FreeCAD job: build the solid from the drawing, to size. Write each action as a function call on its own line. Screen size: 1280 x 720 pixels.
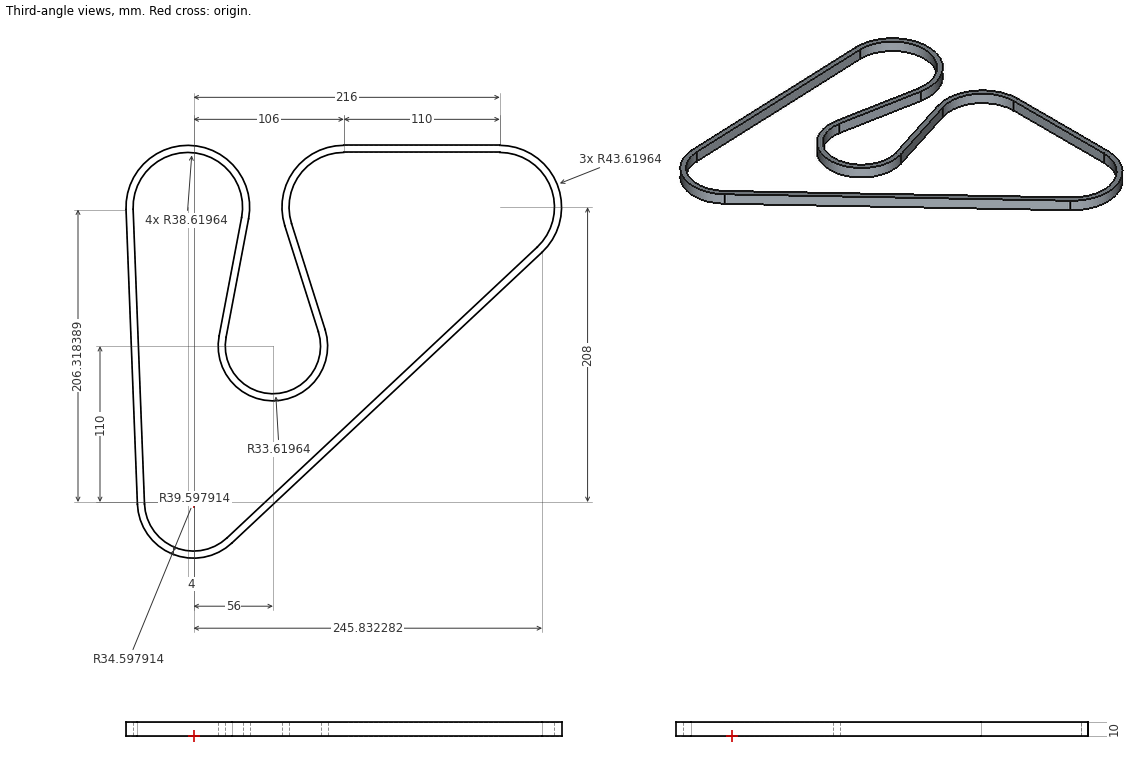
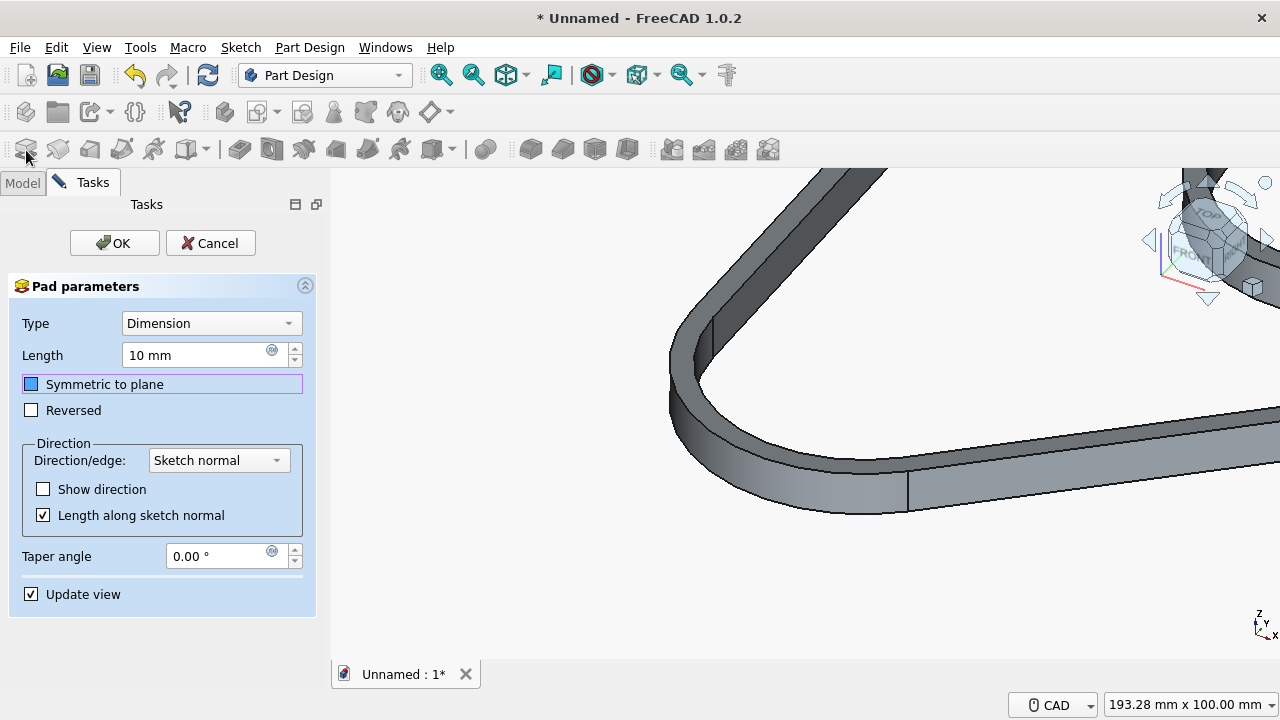
click(115, 243)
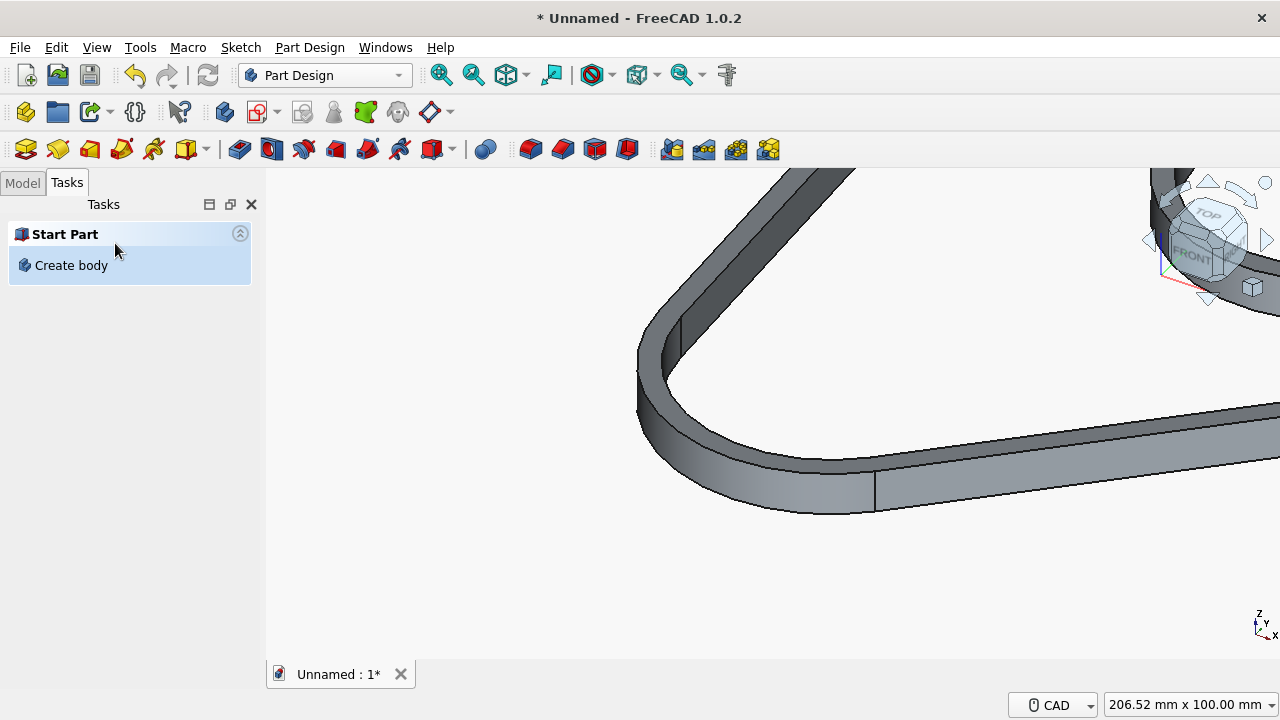
key(0)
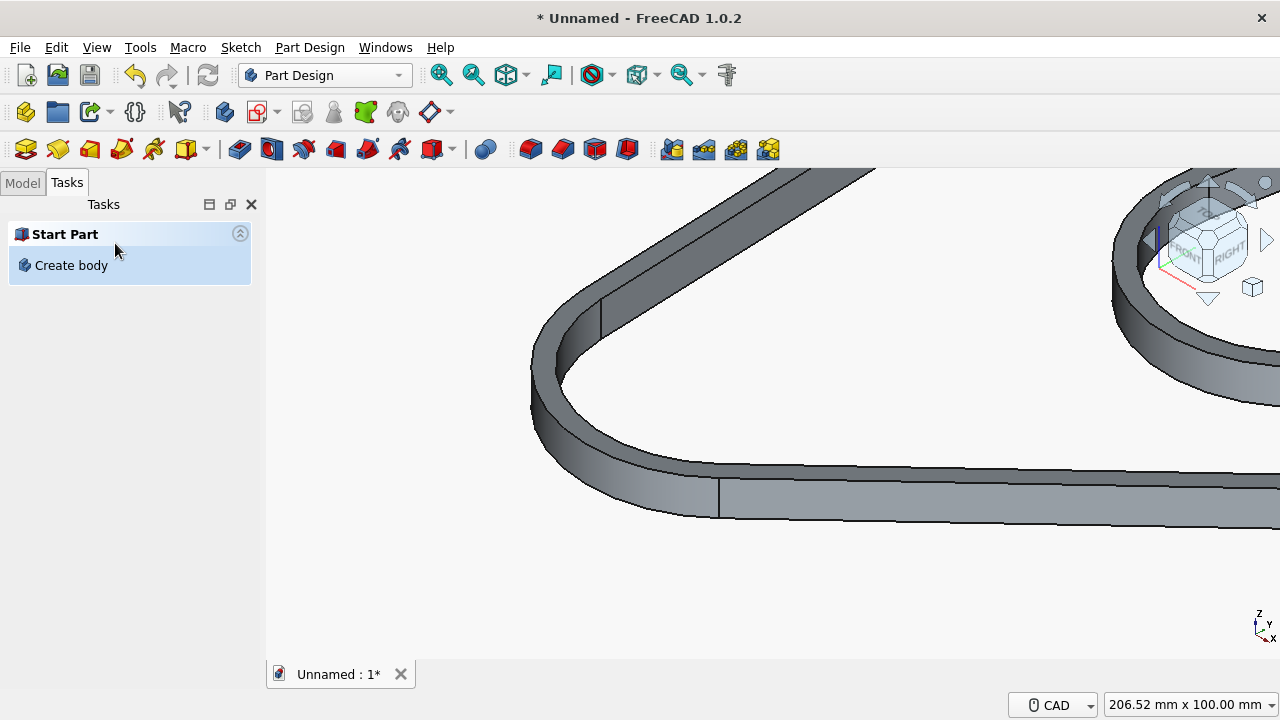
click(442, 76)